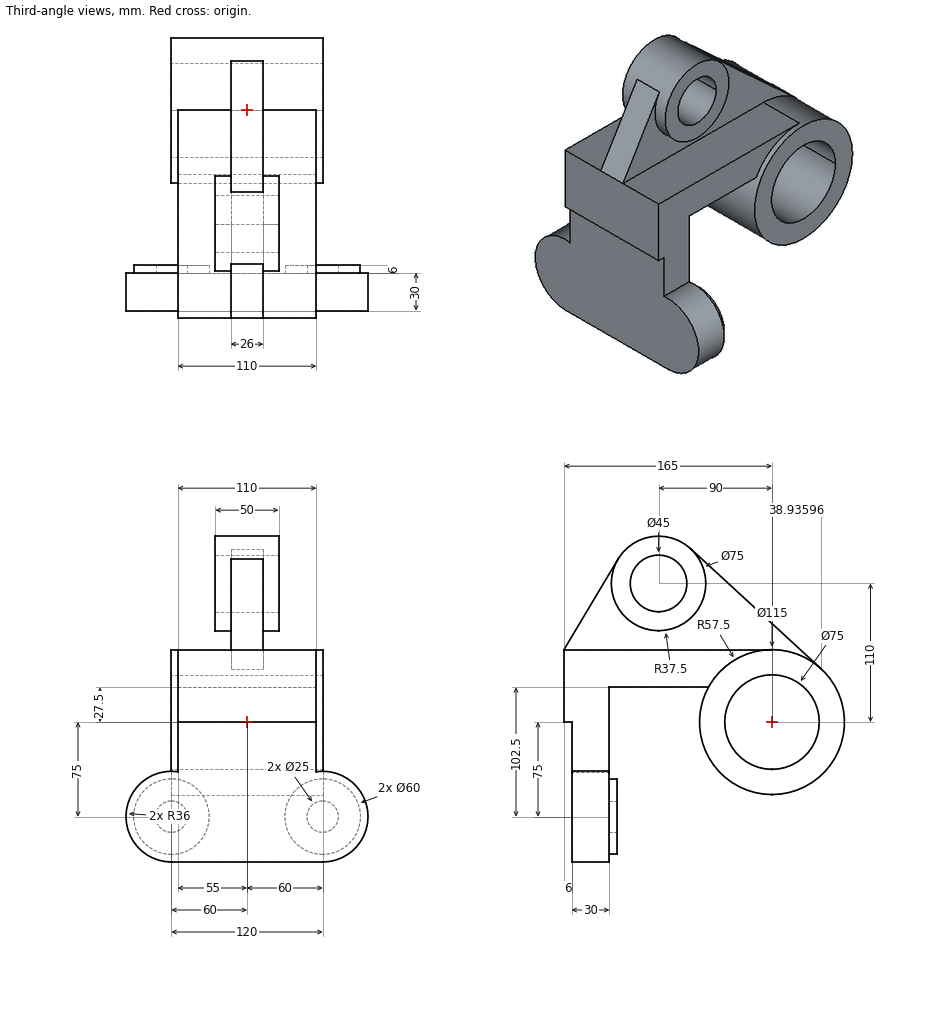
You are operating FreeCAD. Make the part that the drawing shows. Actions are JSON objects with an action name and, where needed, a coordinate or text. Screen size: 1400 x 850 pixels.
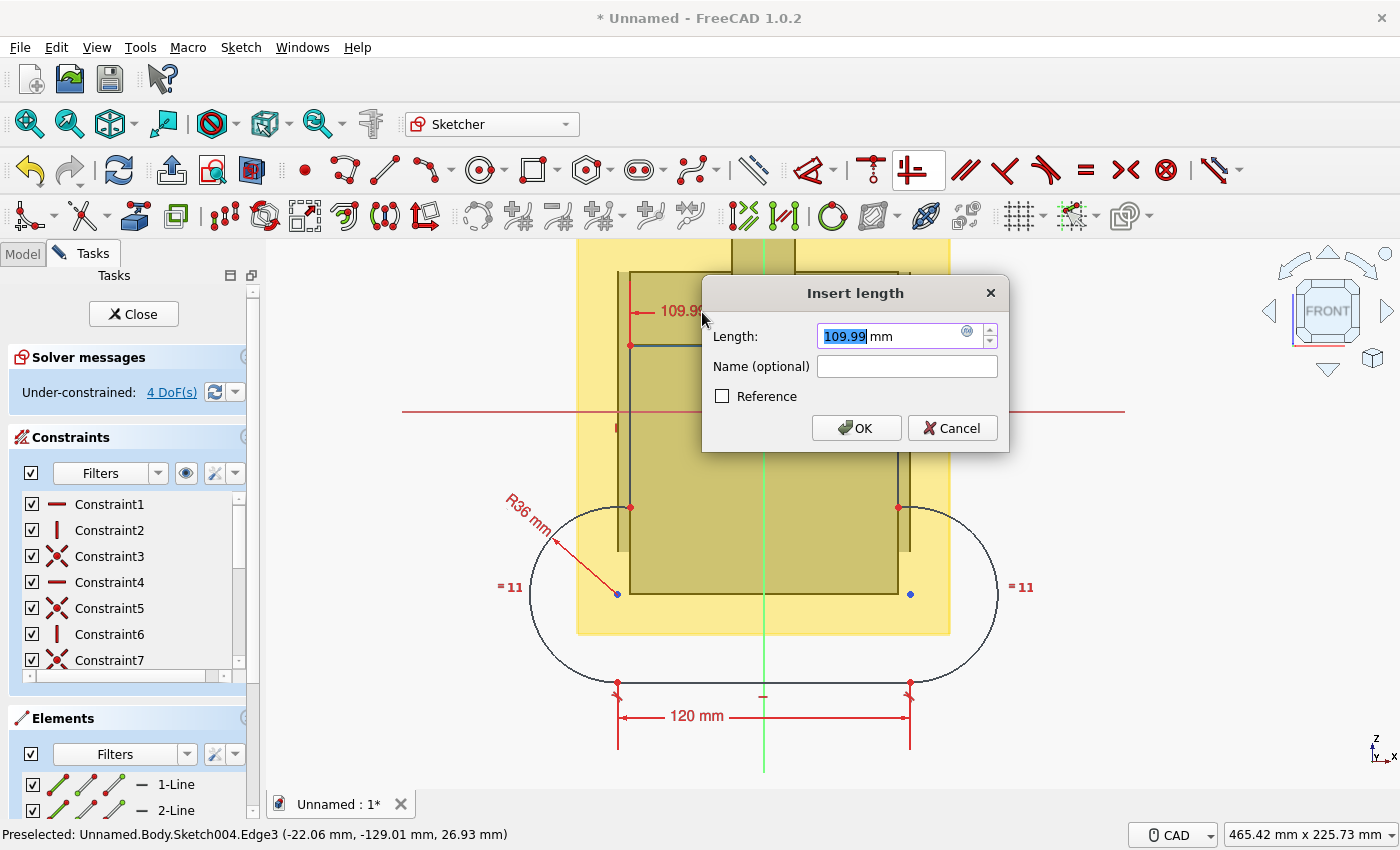
{"action": "type", "text": "110"}
{"action": "key", "text": "Return"}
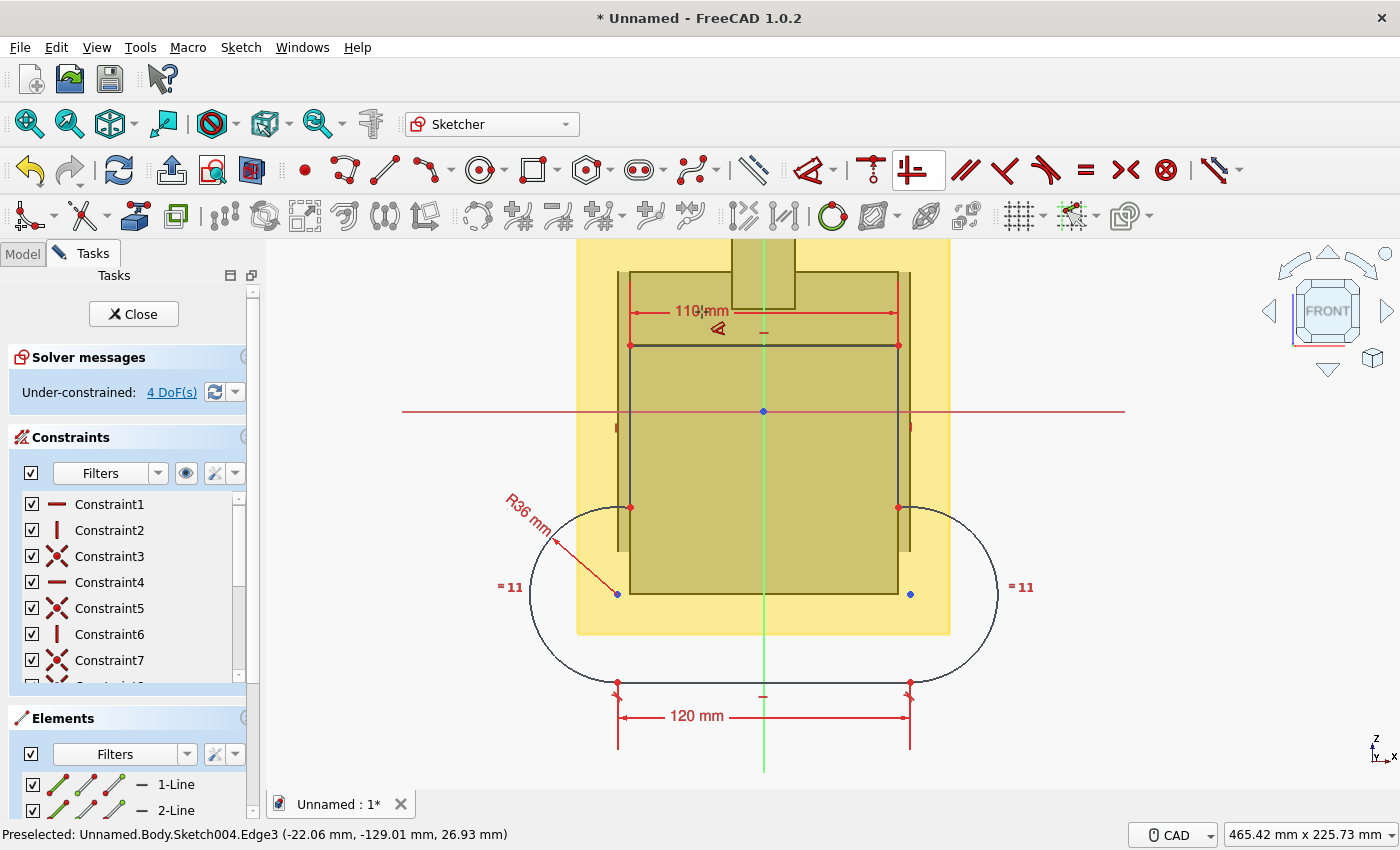
{"action": "left_click", "coordinate": [910, 683]}
{"action": "left_click", "coordinate": [837, 717]}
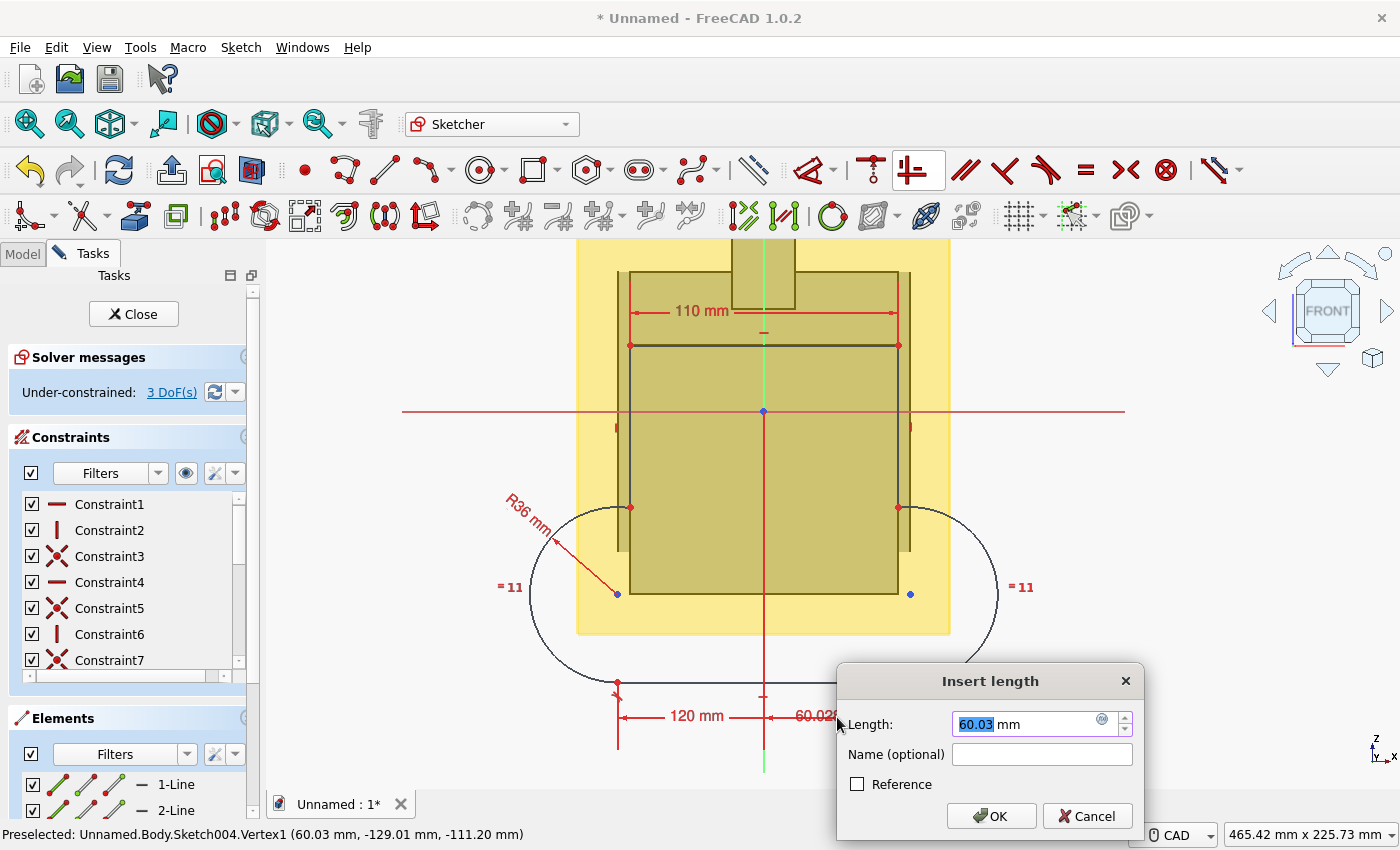
{"action": "type", "text": "60"}
{"action": "key", "text": "Return"}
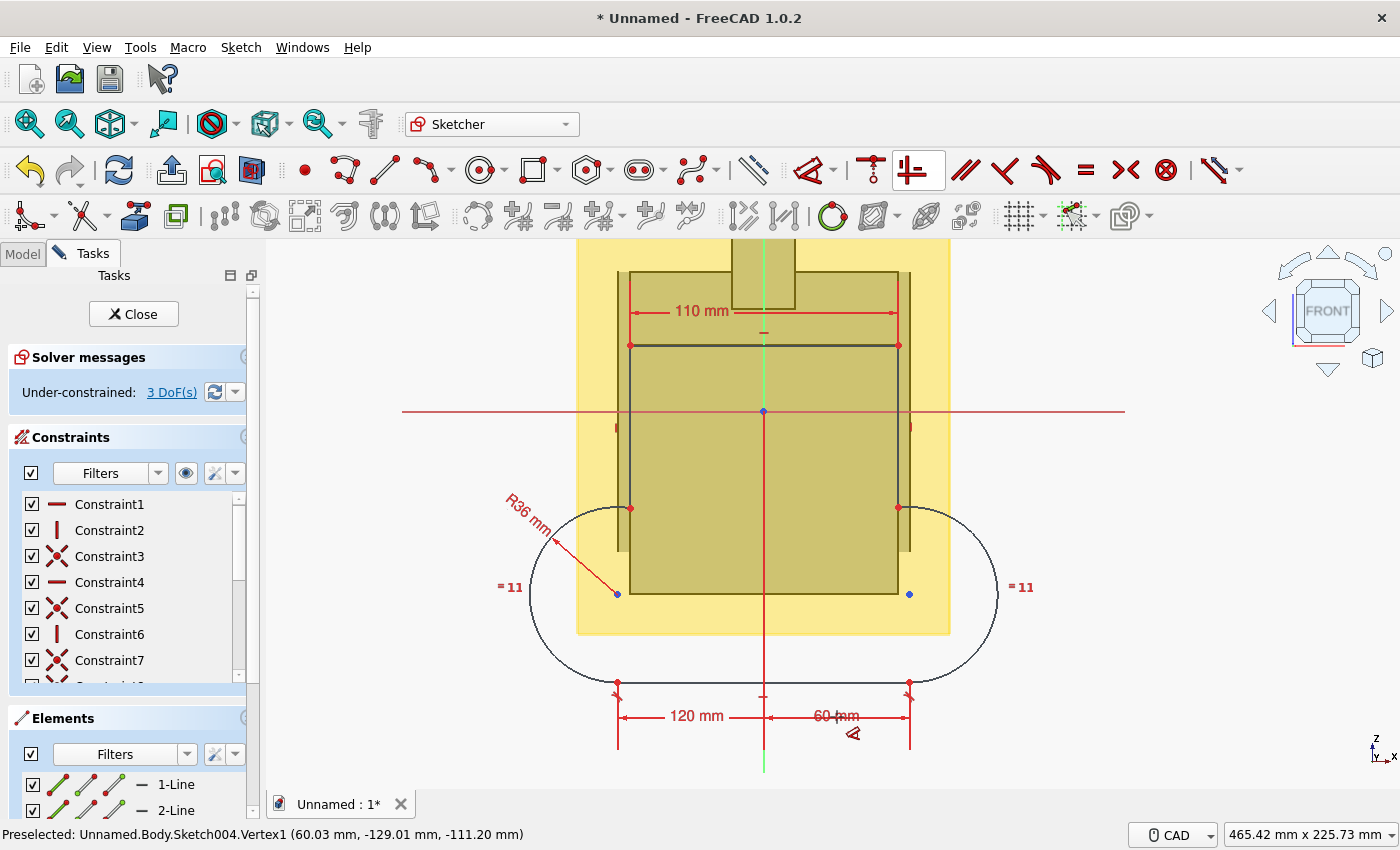
{"action": "left_click", "coordinate": [630, 508]}
{"action": "left_click", "coordinate": [697, 378]}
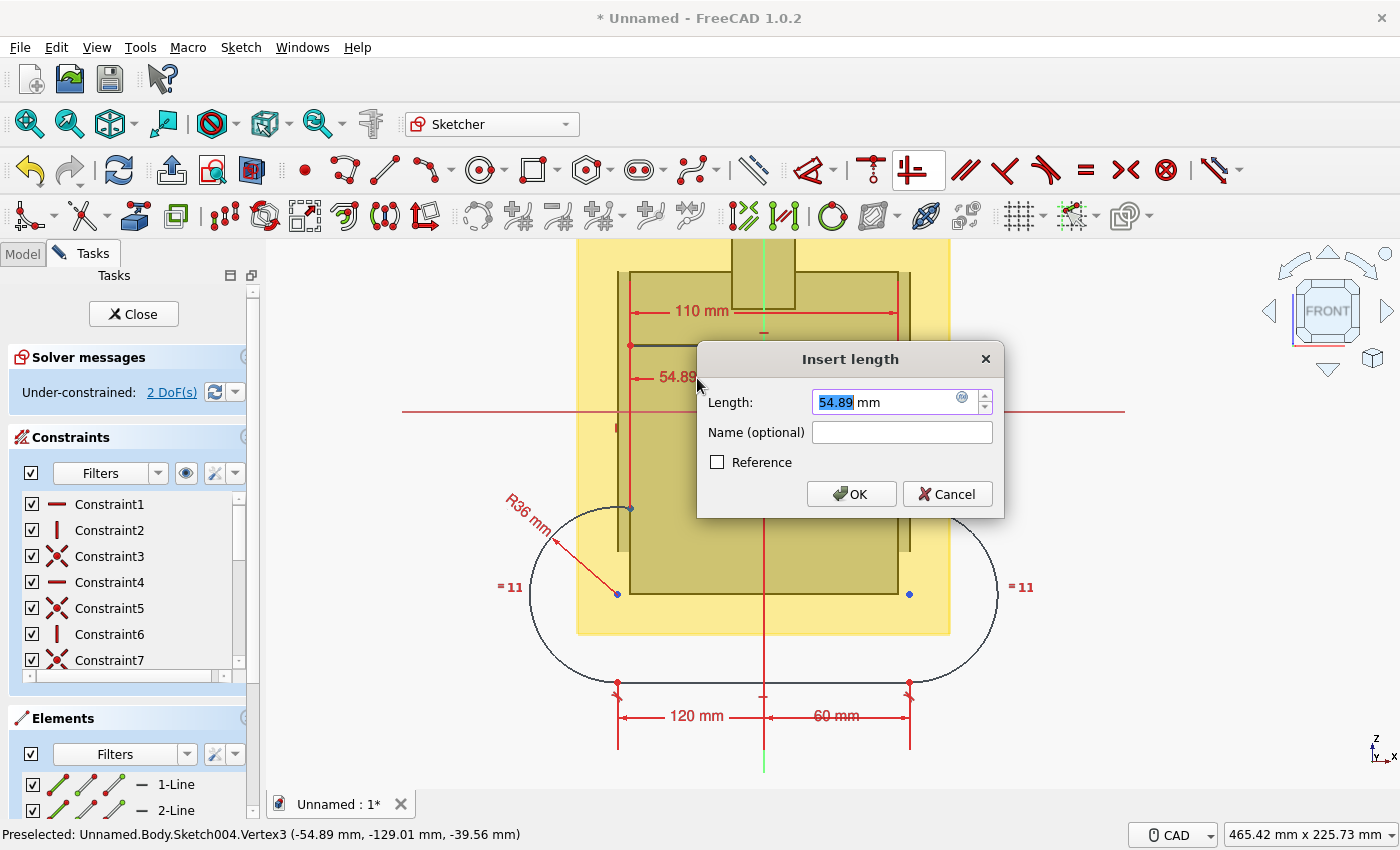
{"action": "type", "text": "55"}
{"action": "key", "text": "Return"}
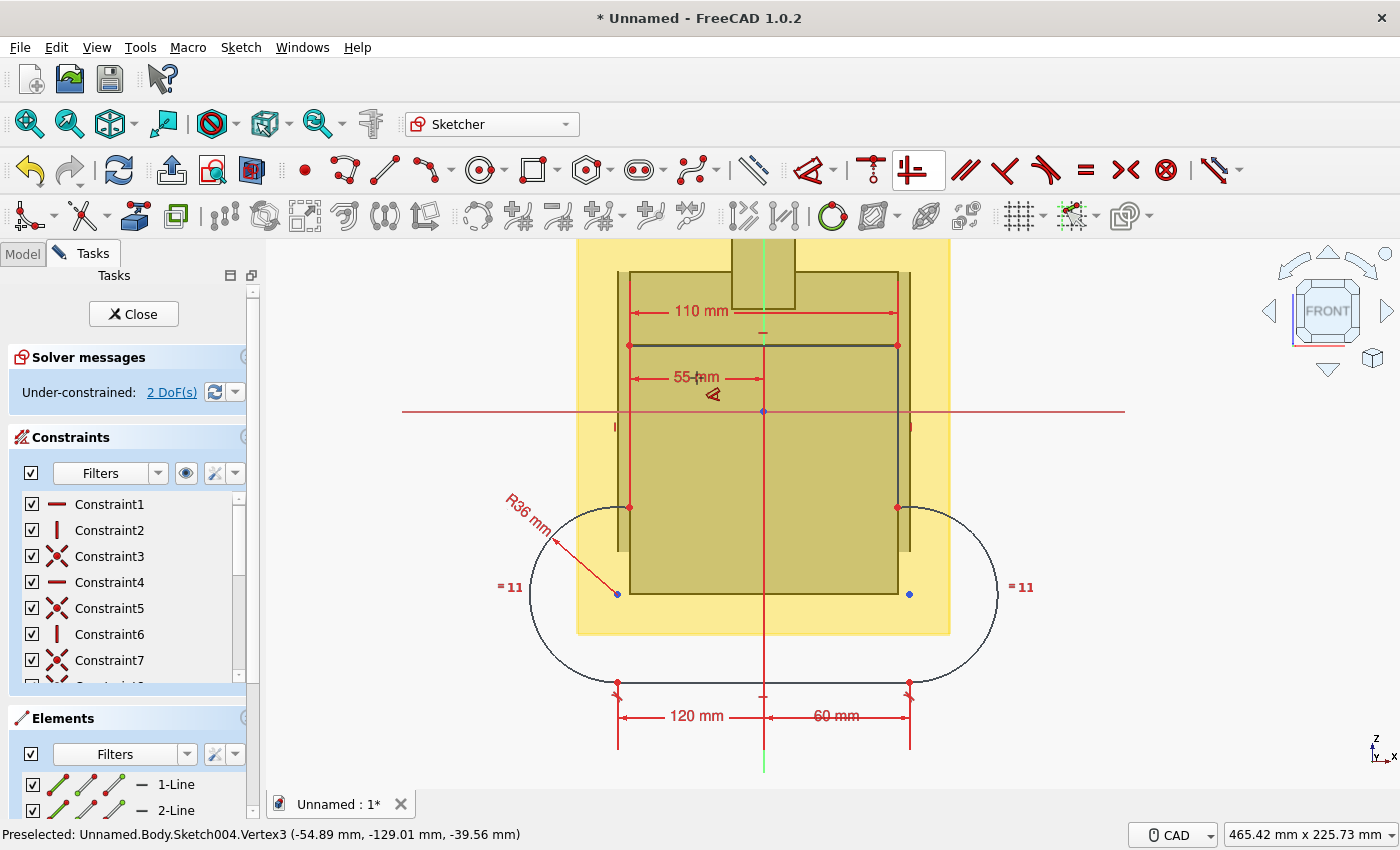
{"action": "left_click", "coordinate": [618, 595]}
{"action": "left_click", "coordinate": [584, 461]}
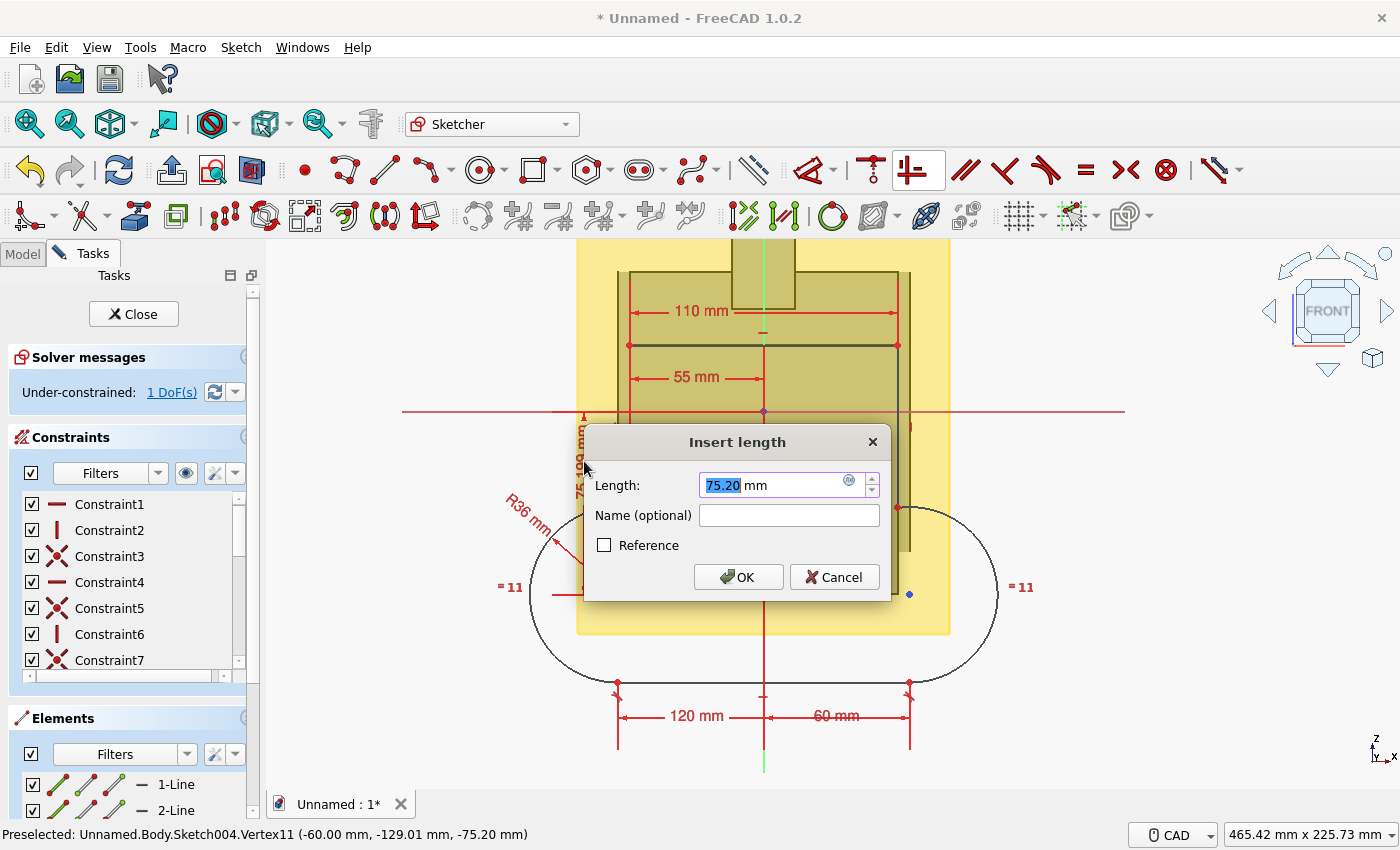
{"action": "type", "text": "75"}
{"action": "key", "text": "Return"}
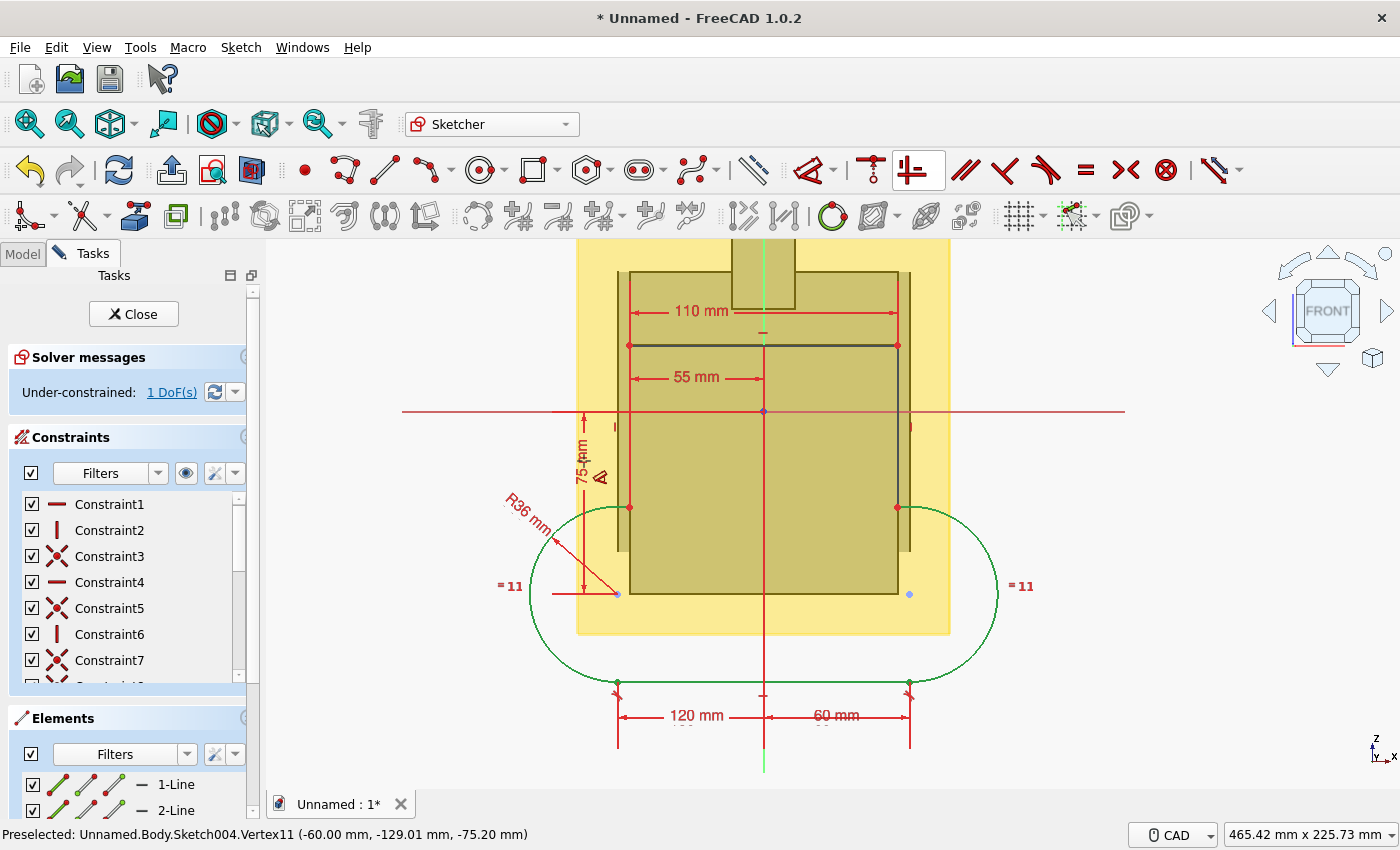
{"action": "left_click", "coordinate": [630, 346]}
{"action": "left_click", "coordinate": [596, 379]}